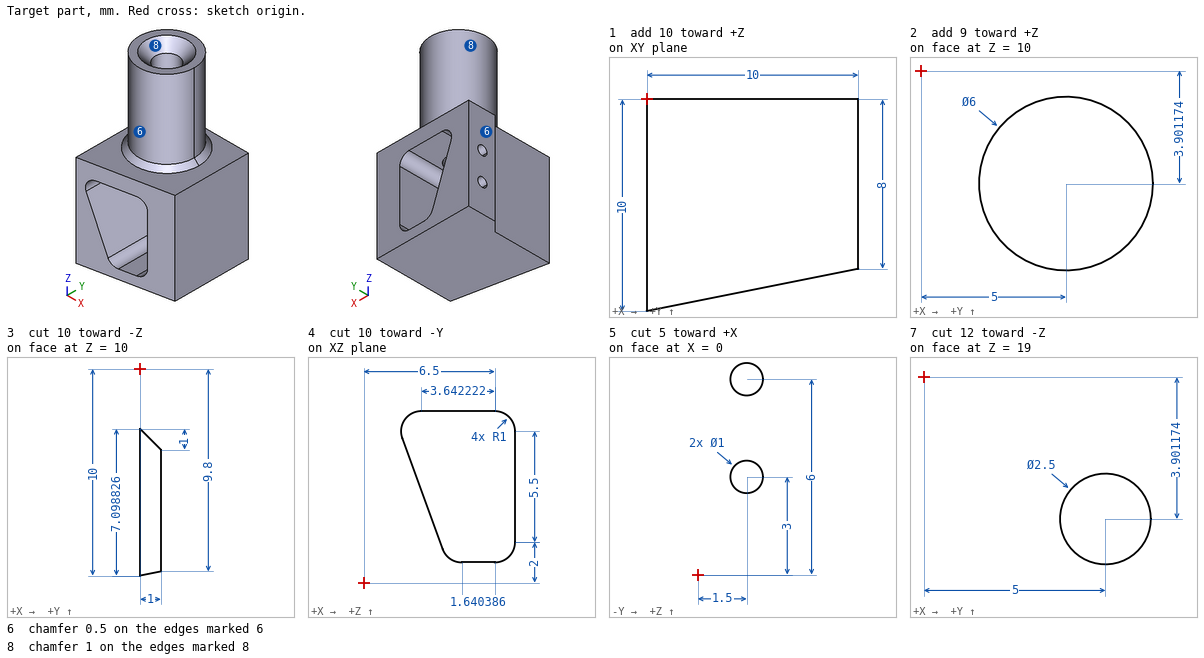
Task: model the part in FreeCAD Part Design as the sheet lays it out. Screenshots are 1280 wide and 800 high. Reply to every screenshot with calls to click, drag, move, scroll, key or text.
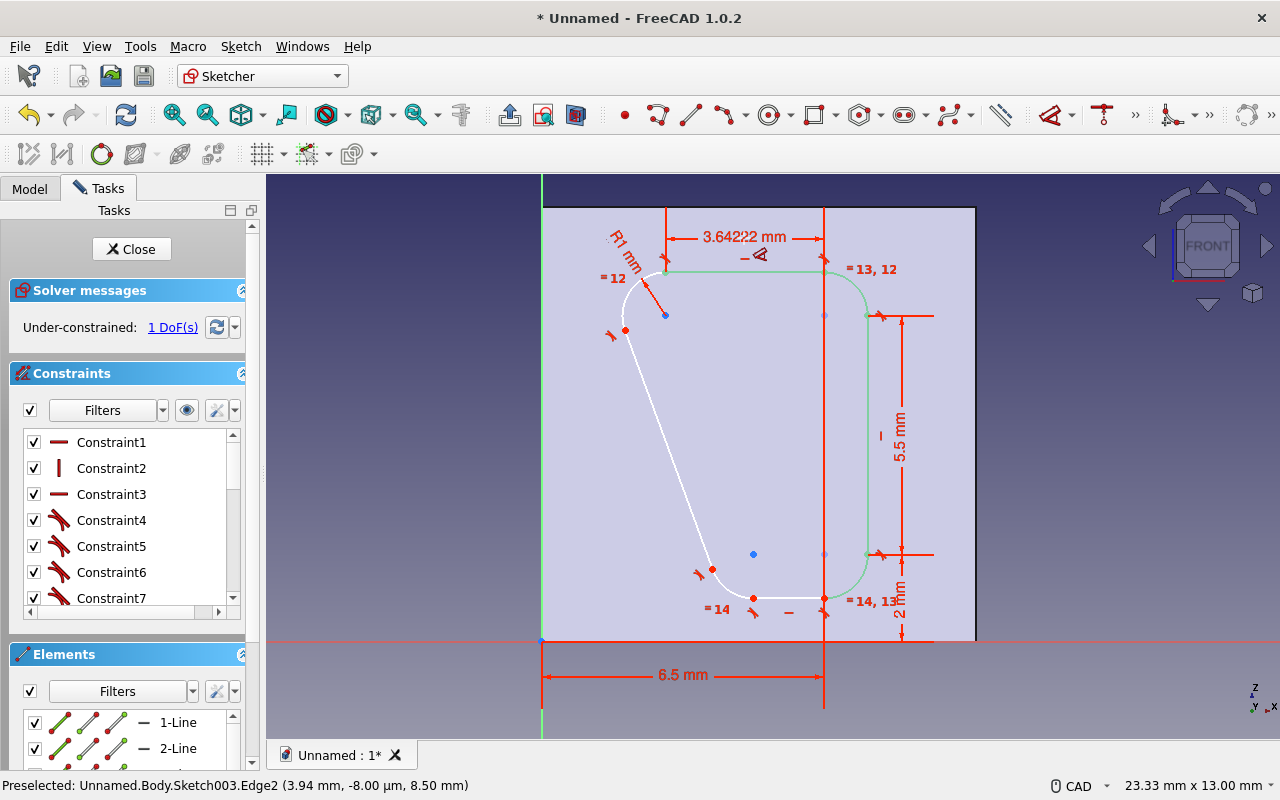
click(803, 598)
click(789, 564)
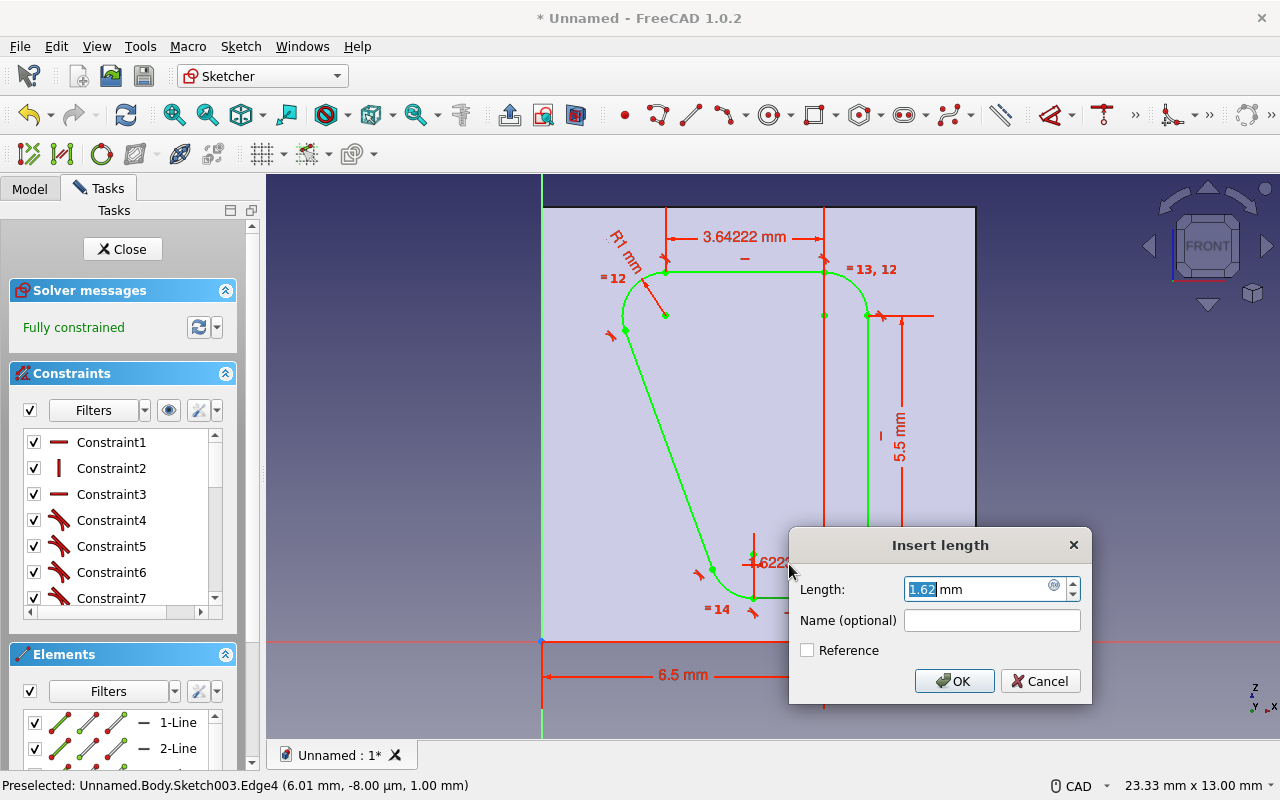
text(1.640386)
key(Return)
key(Escape)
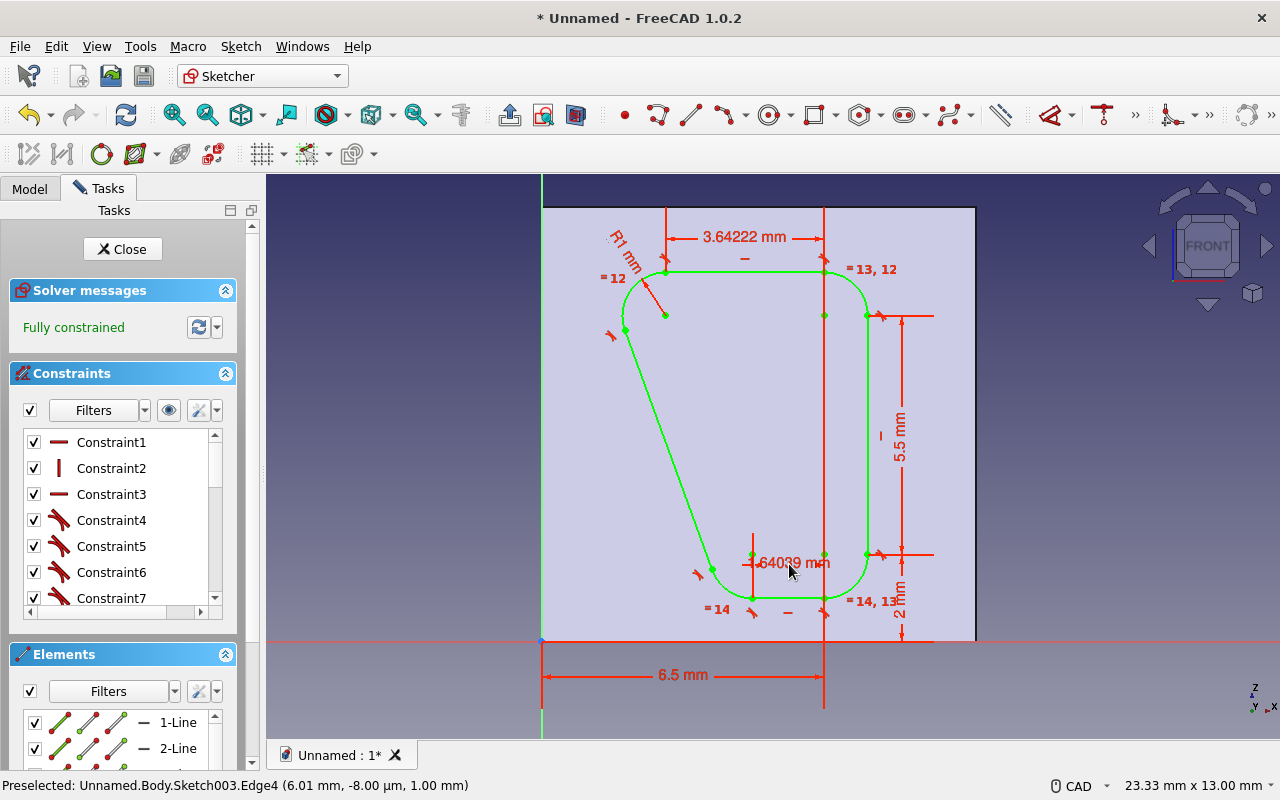
click(123, 249)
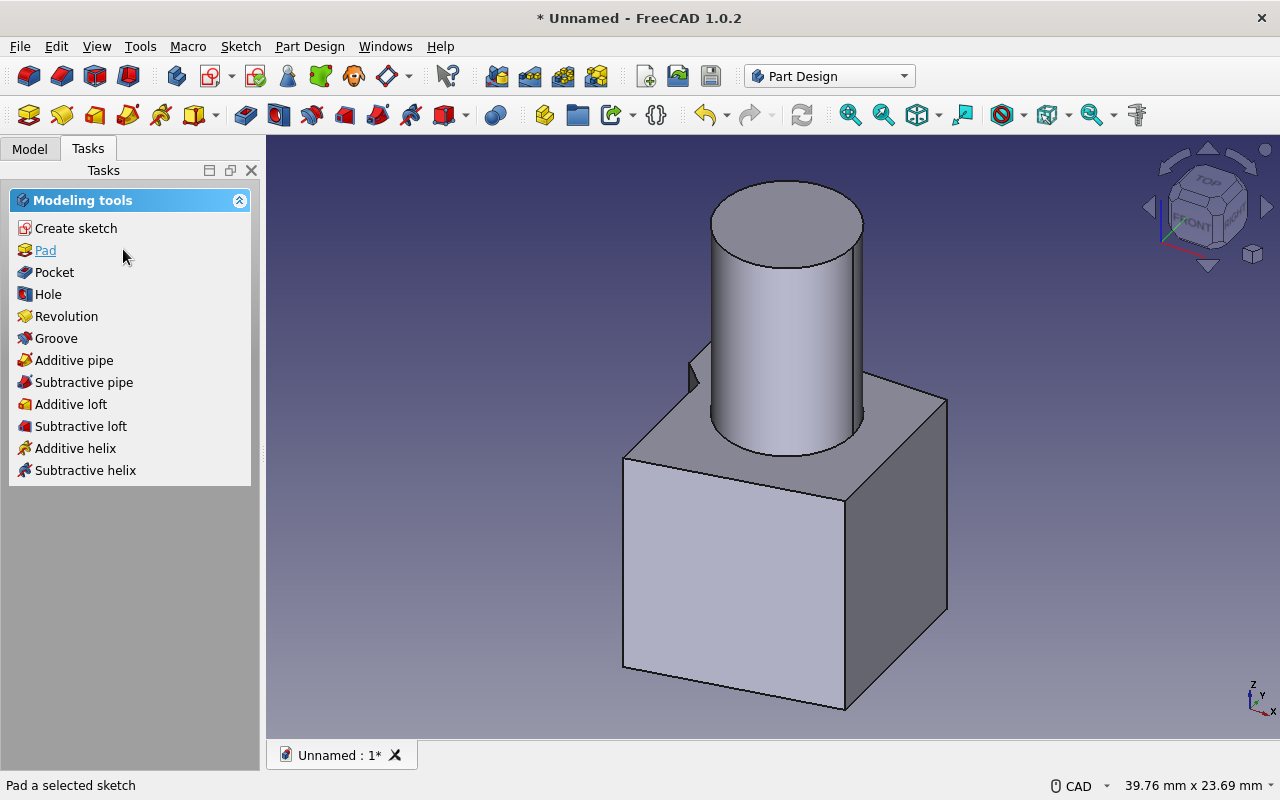
click(246, 116)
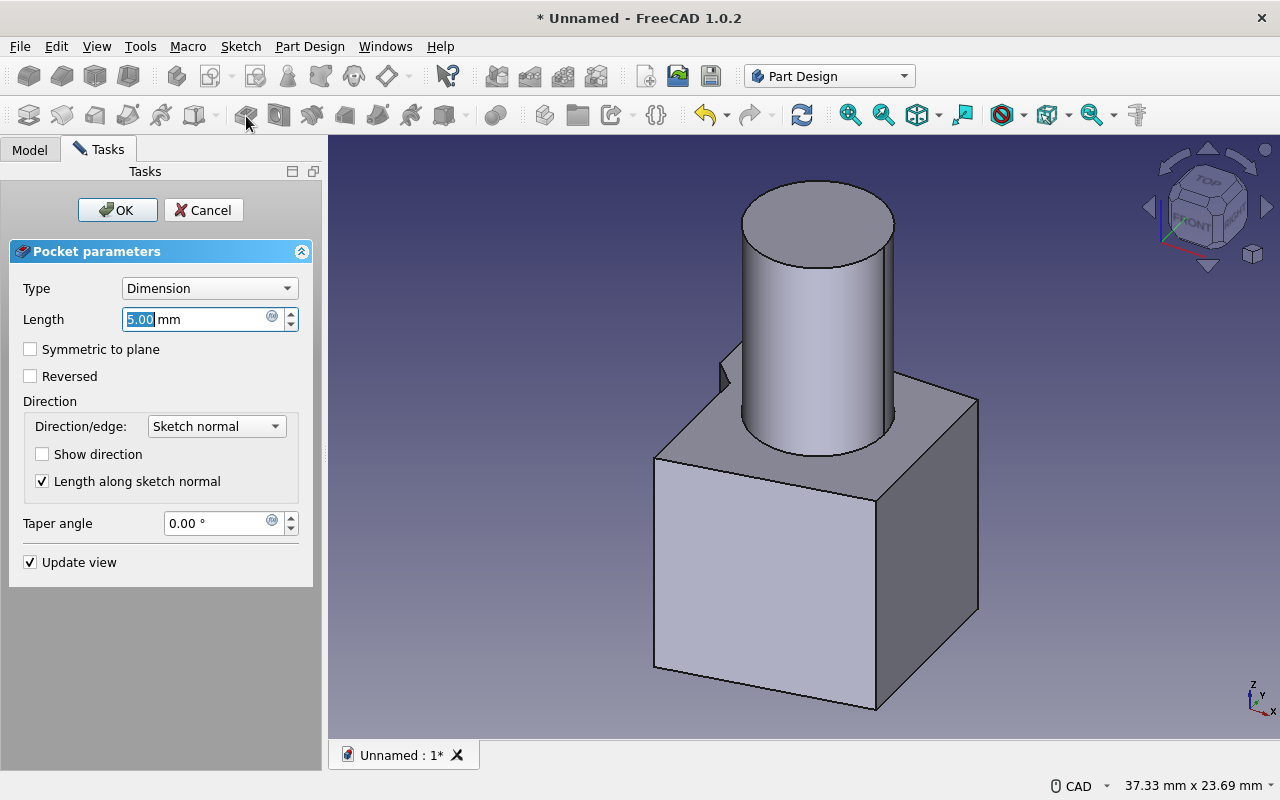
text(10)
key(Tab)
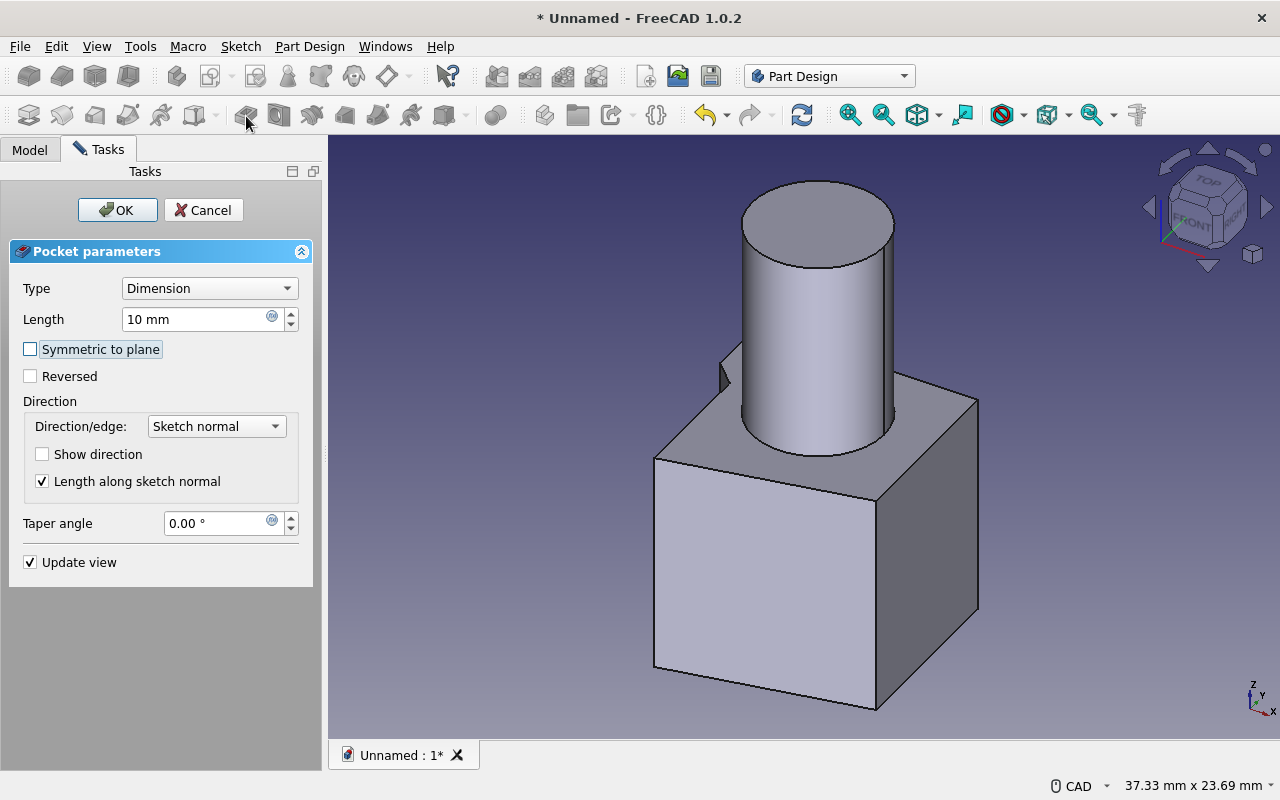
click(31, 376)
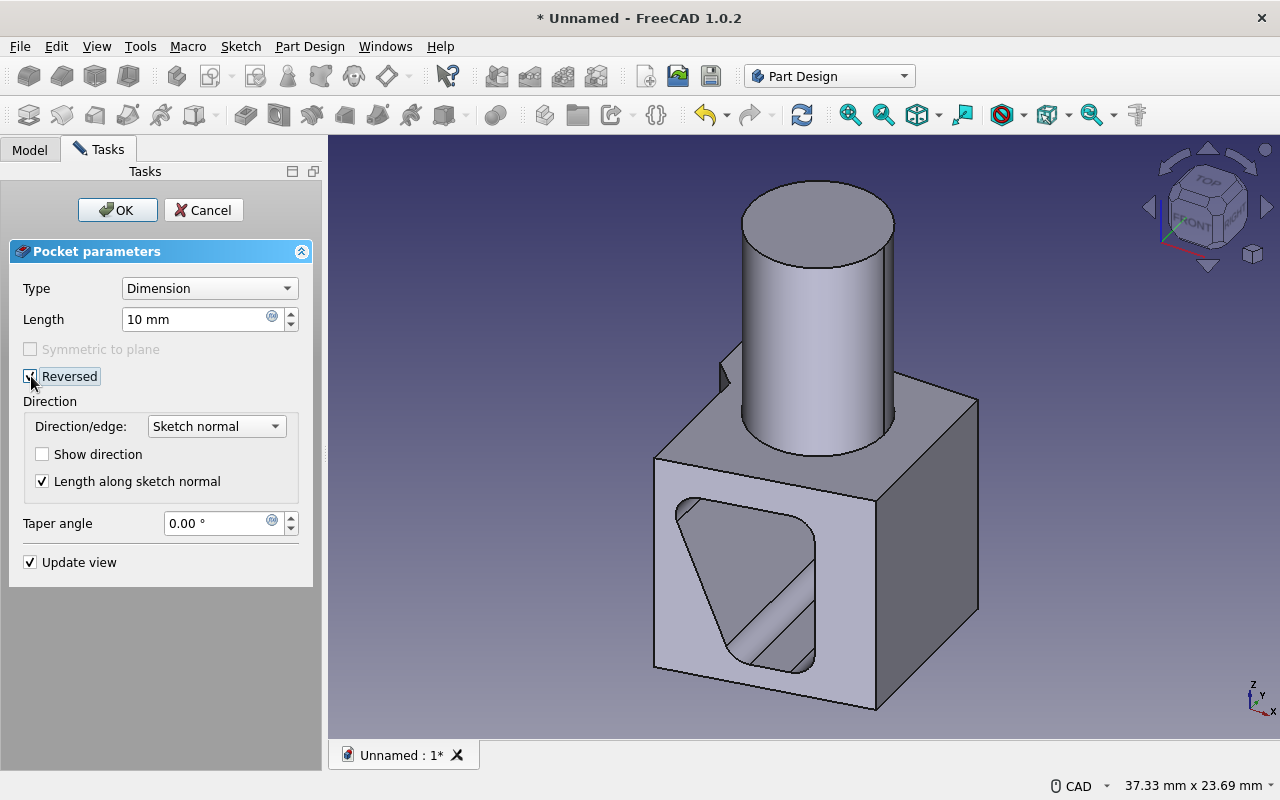
click(118, 210)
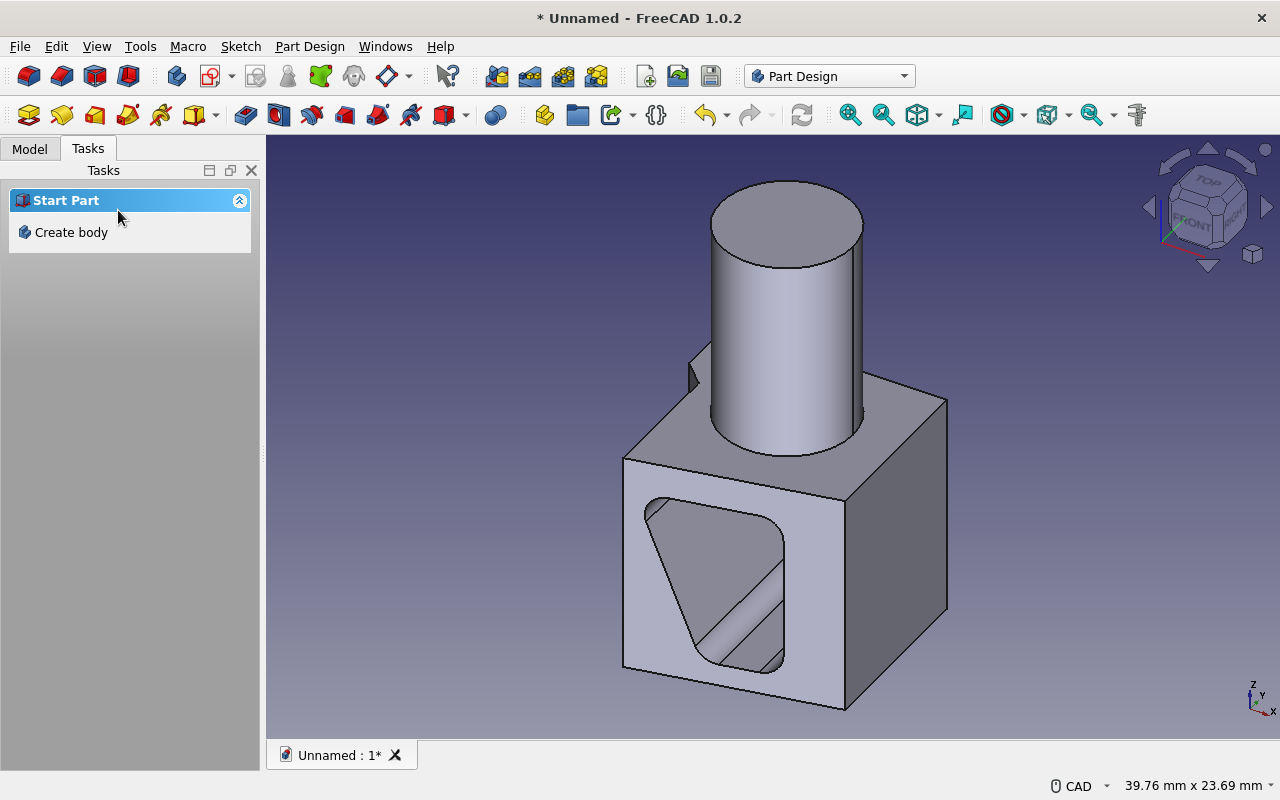
key(6)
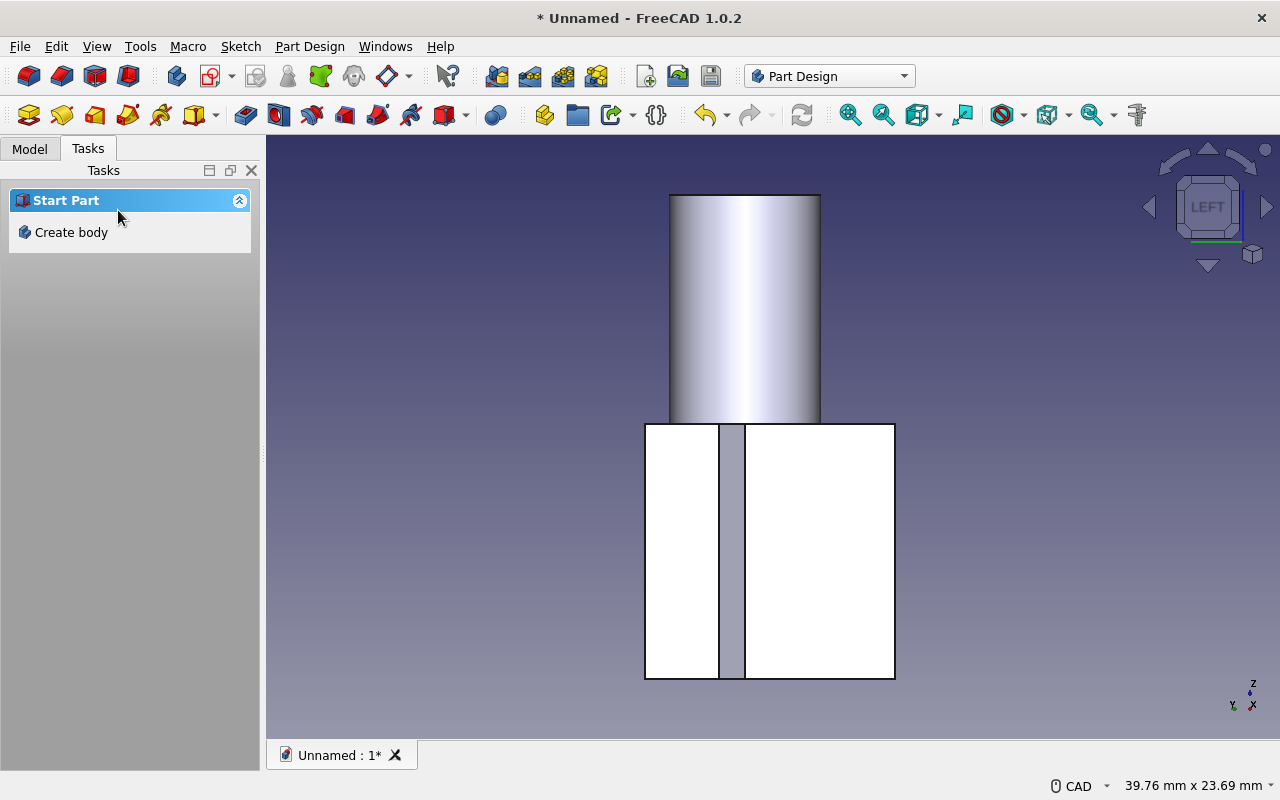
click(682, 478)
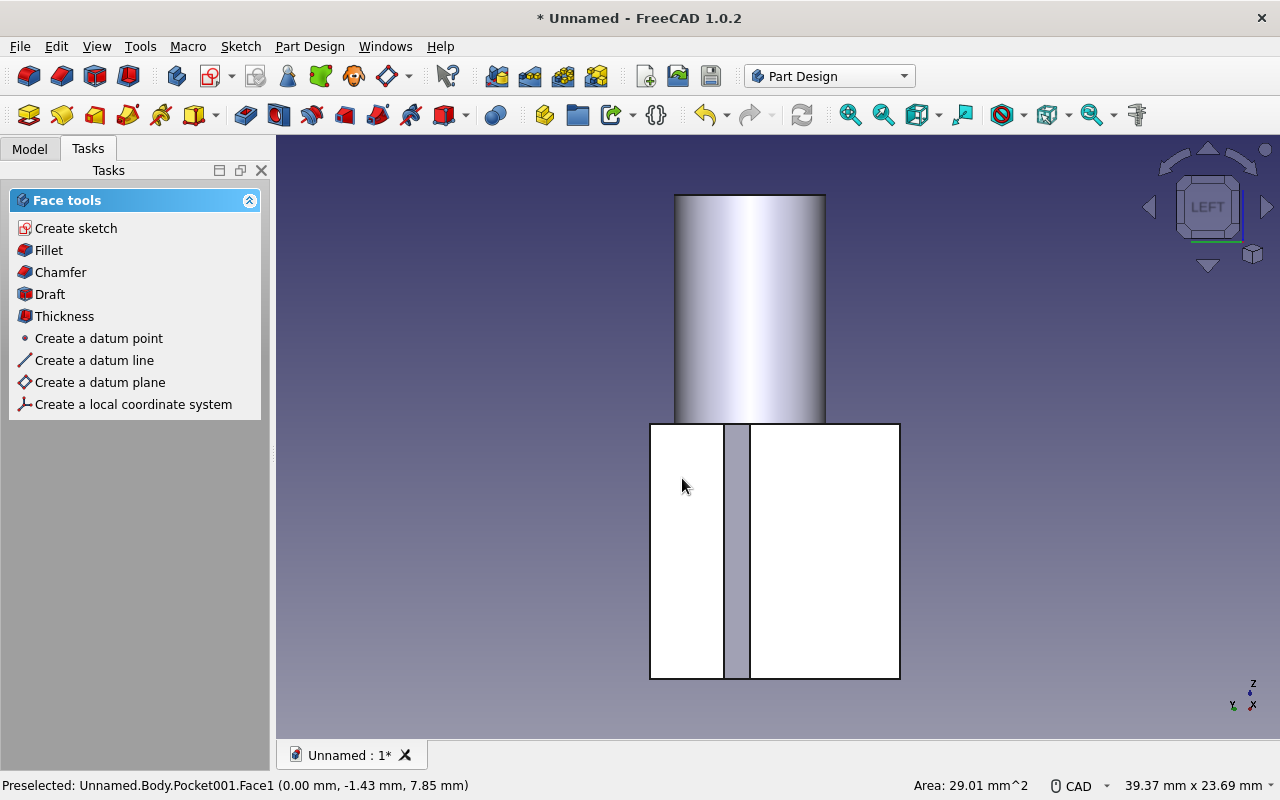
click(210, 76)